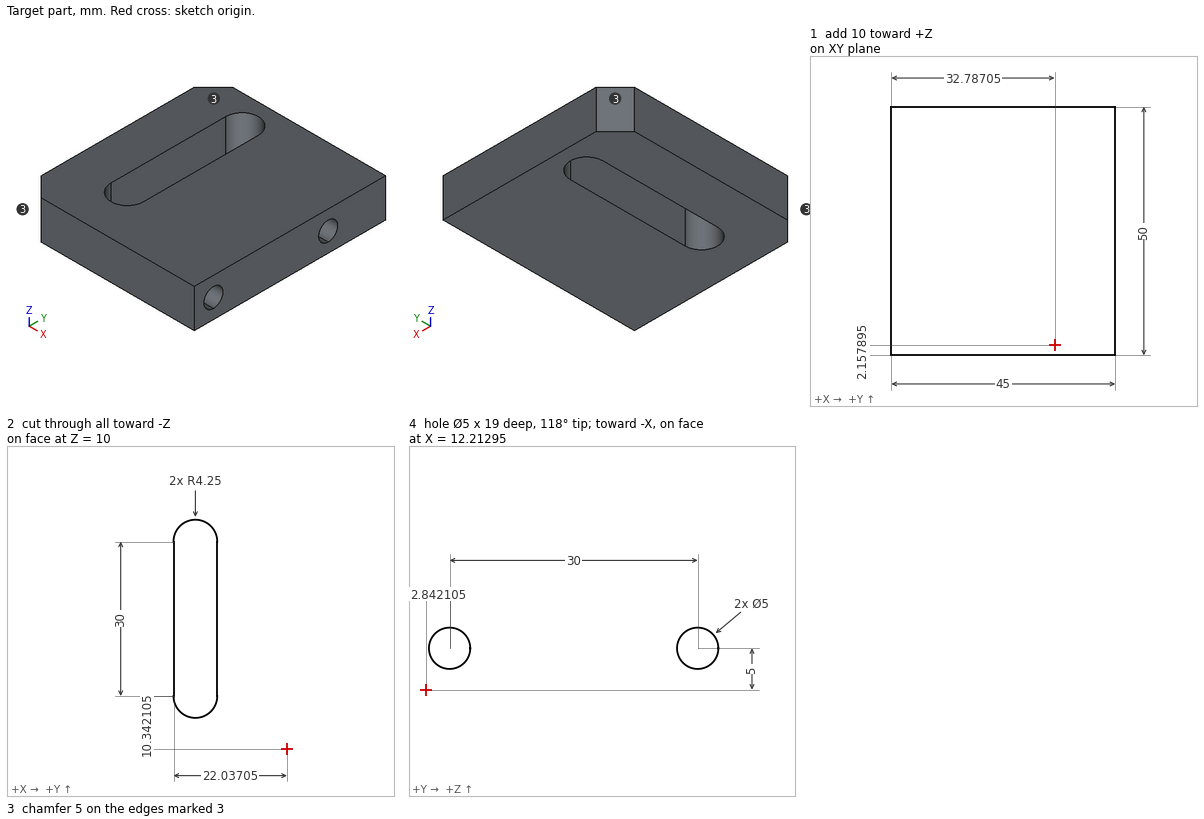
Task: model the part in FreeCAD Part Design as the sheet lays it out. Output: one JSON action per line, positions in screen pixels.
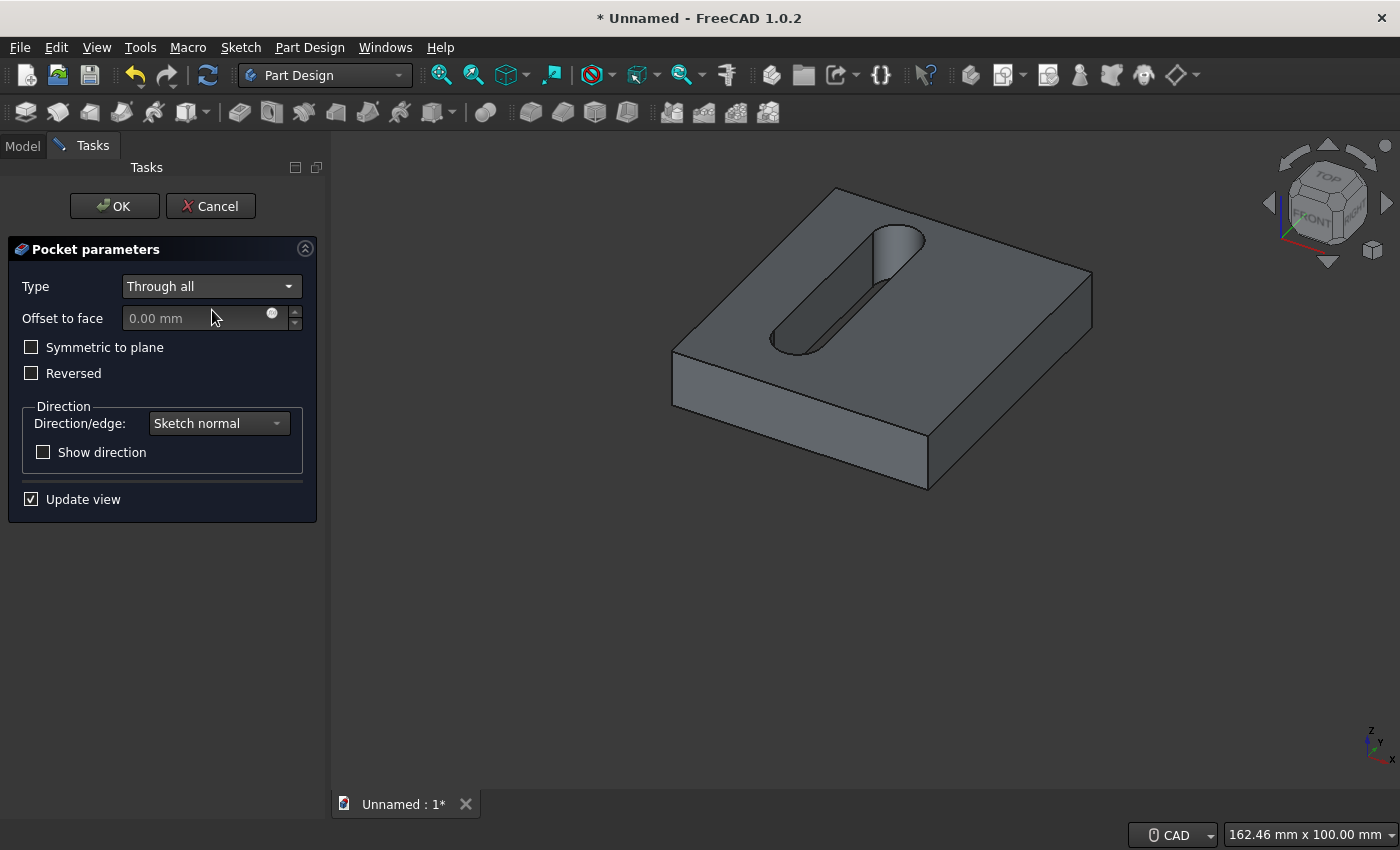
{"action": "left_click", "coordinate": [115, 206]}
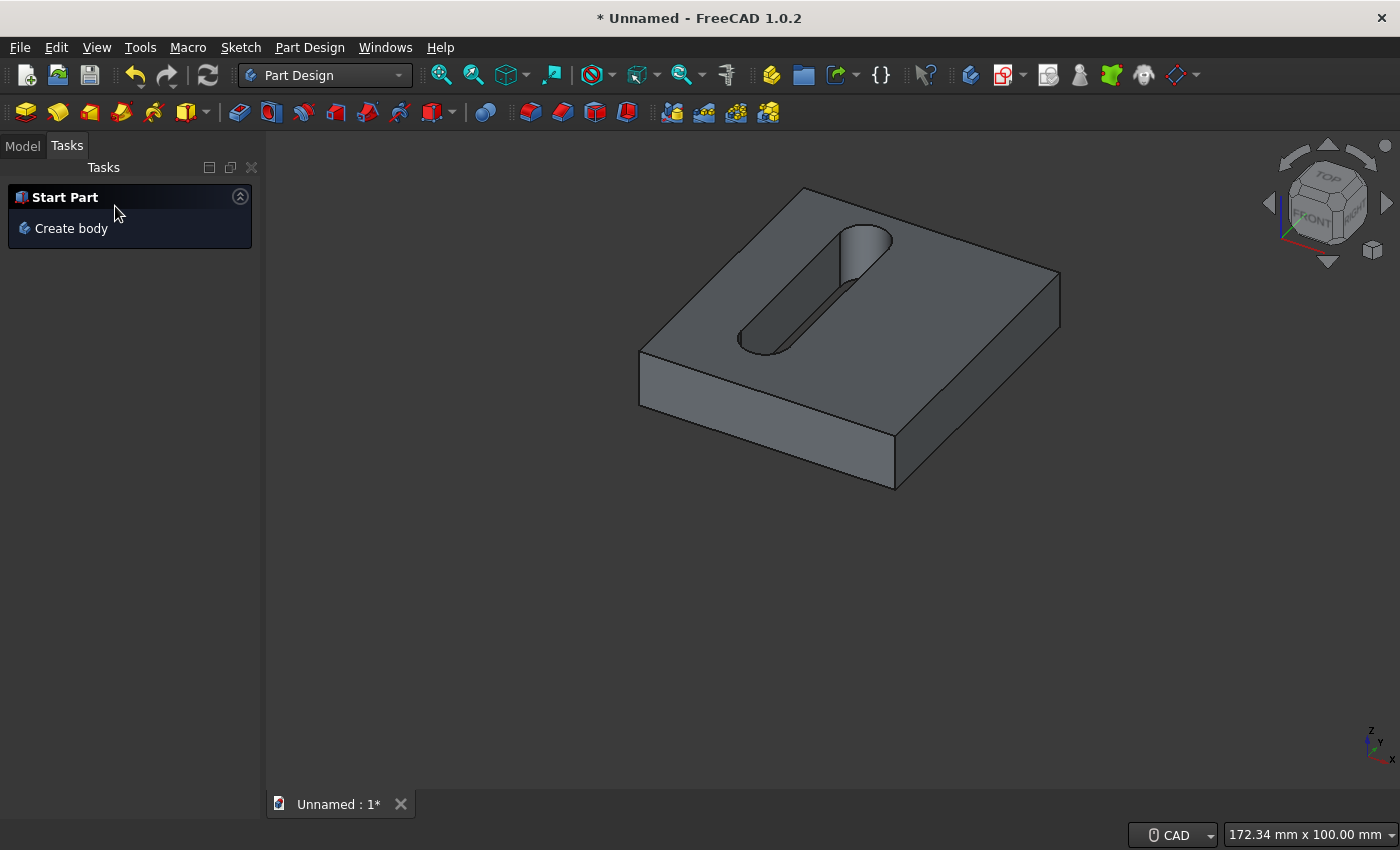
{"action": "key", "text": "0"}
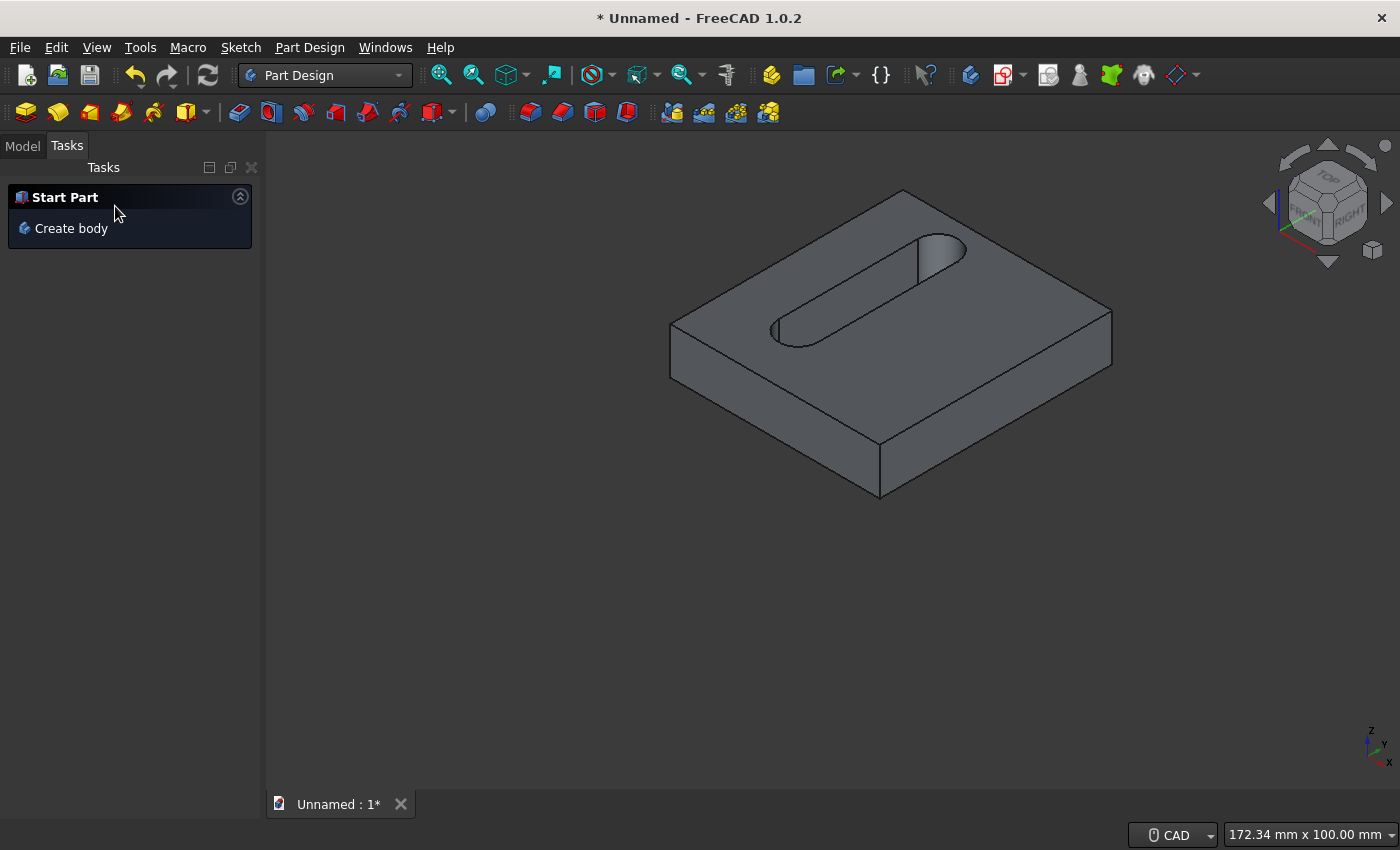
{"action": "key", "text": "2"}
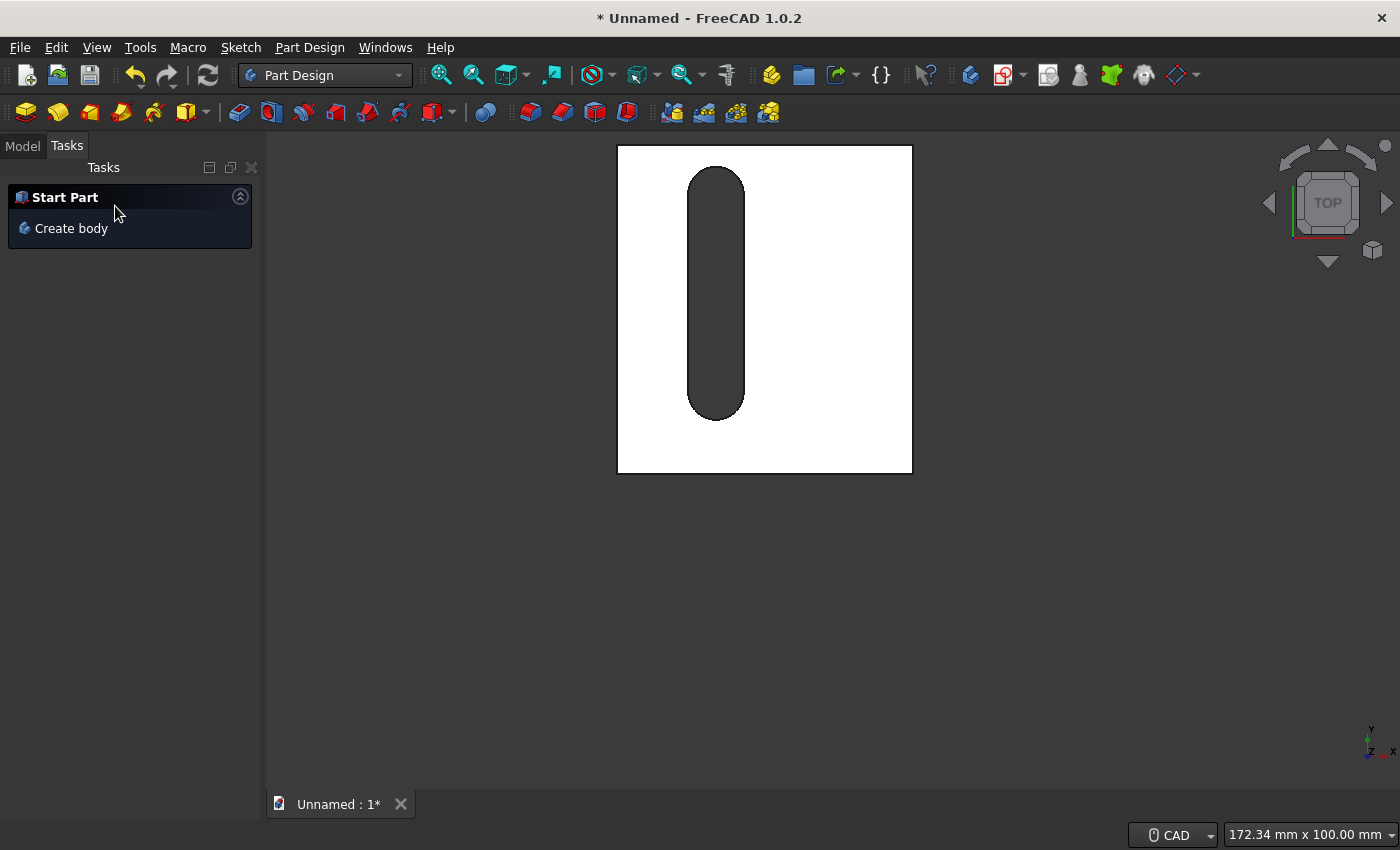
{"action": "key", "text": "1"}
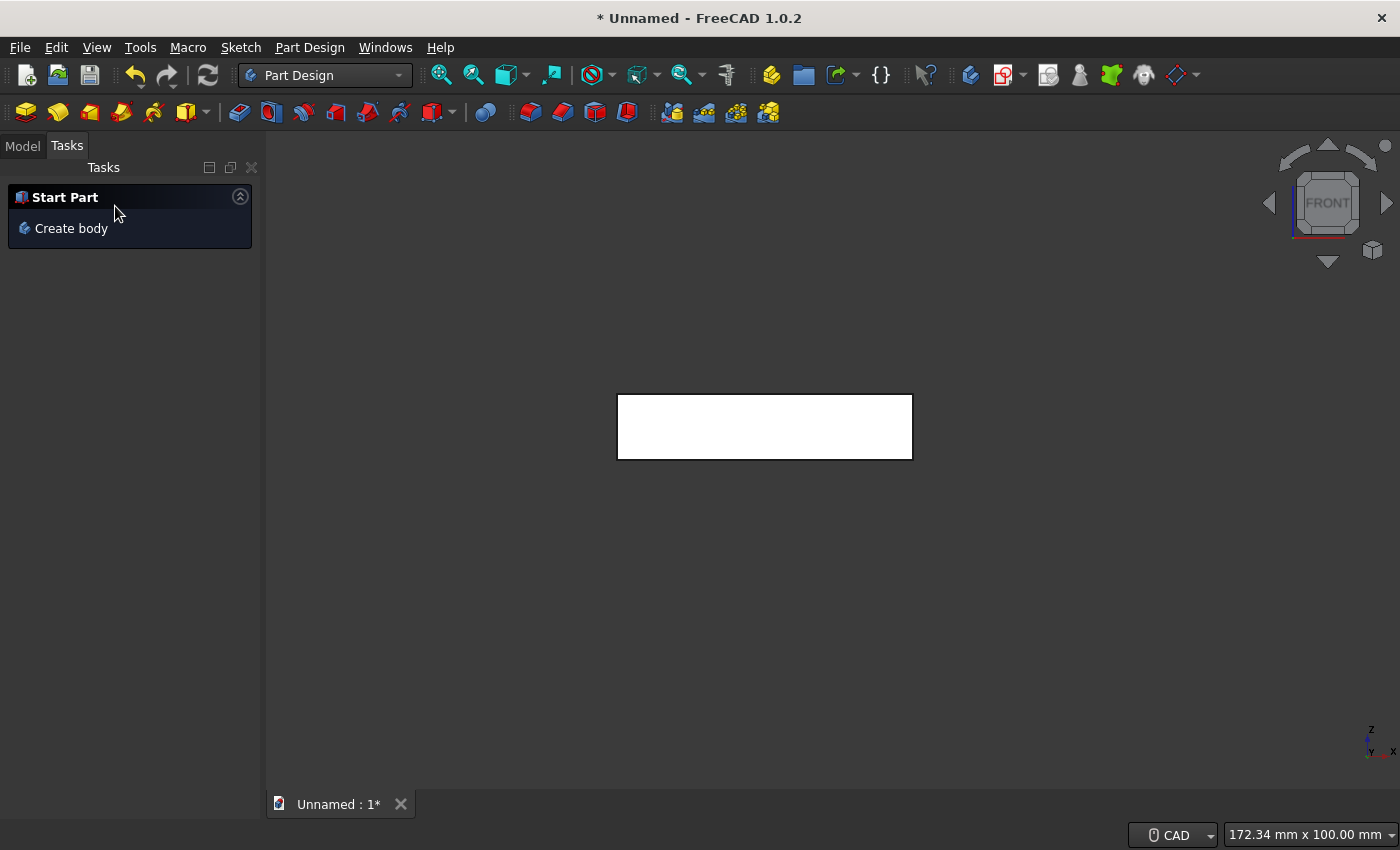
{"action": "left_click", "coordinate": [442, 76]}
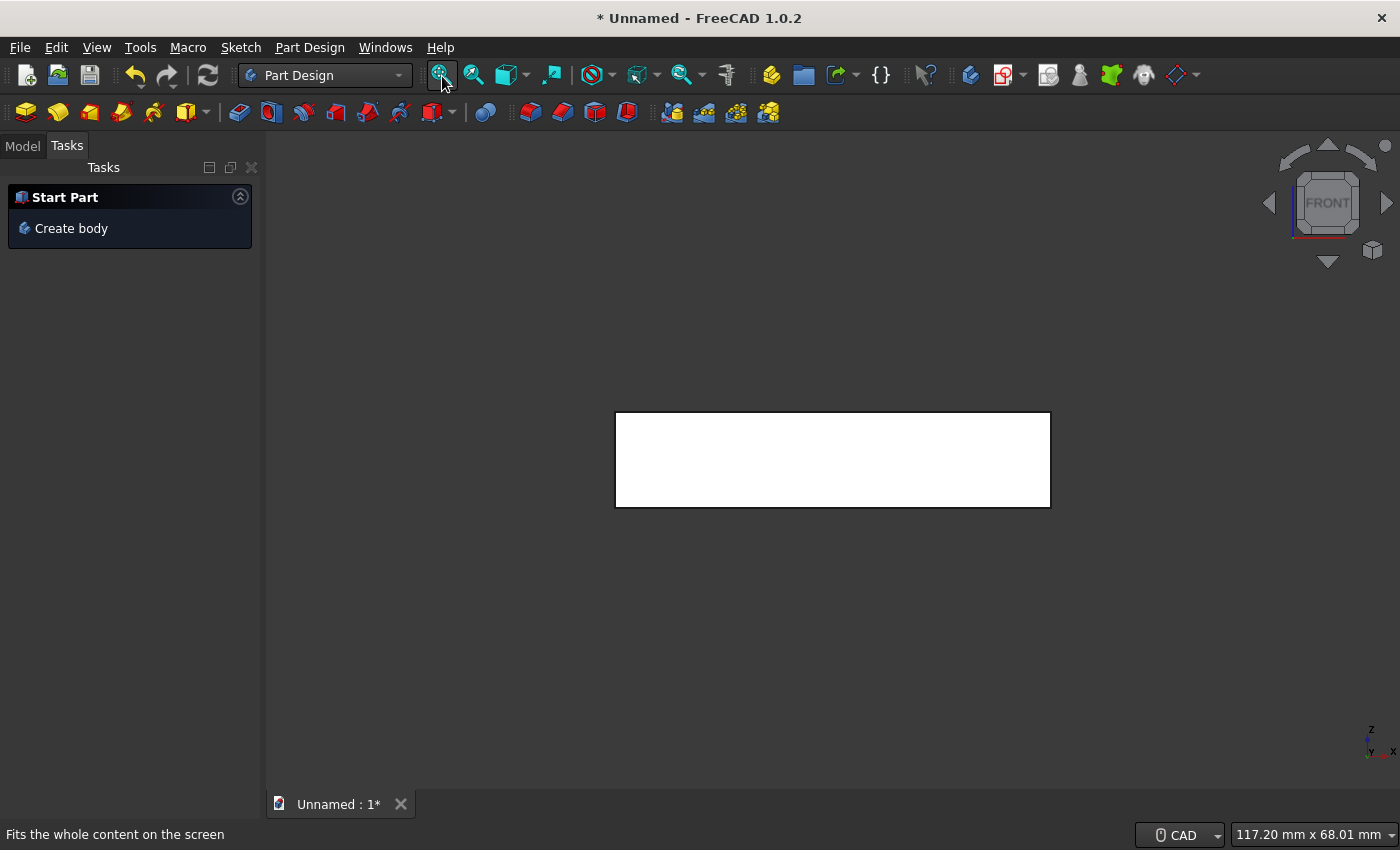
{"action": "left_click", "coordinate": [615, 459]}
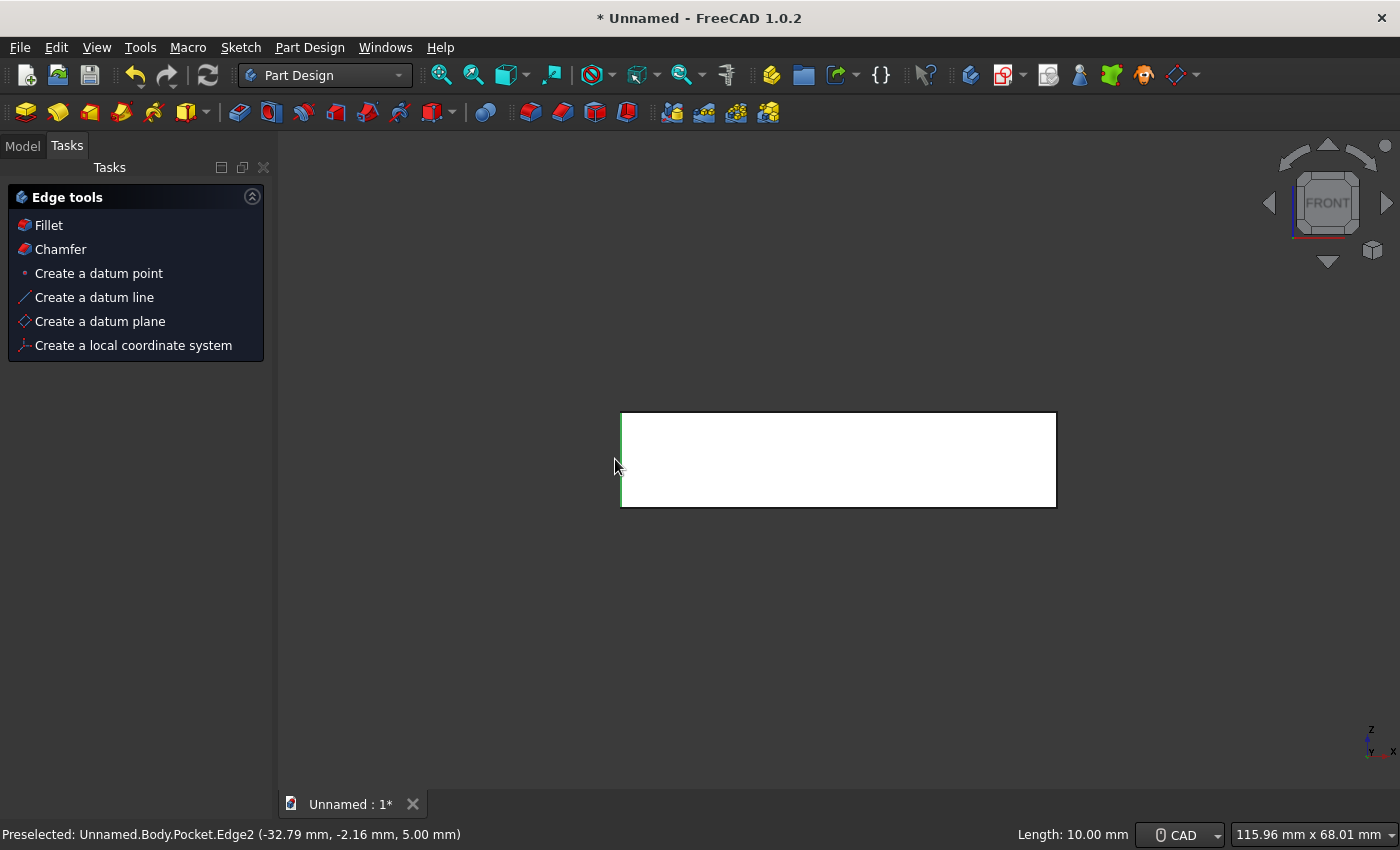
{"action": "key", "text": "3"}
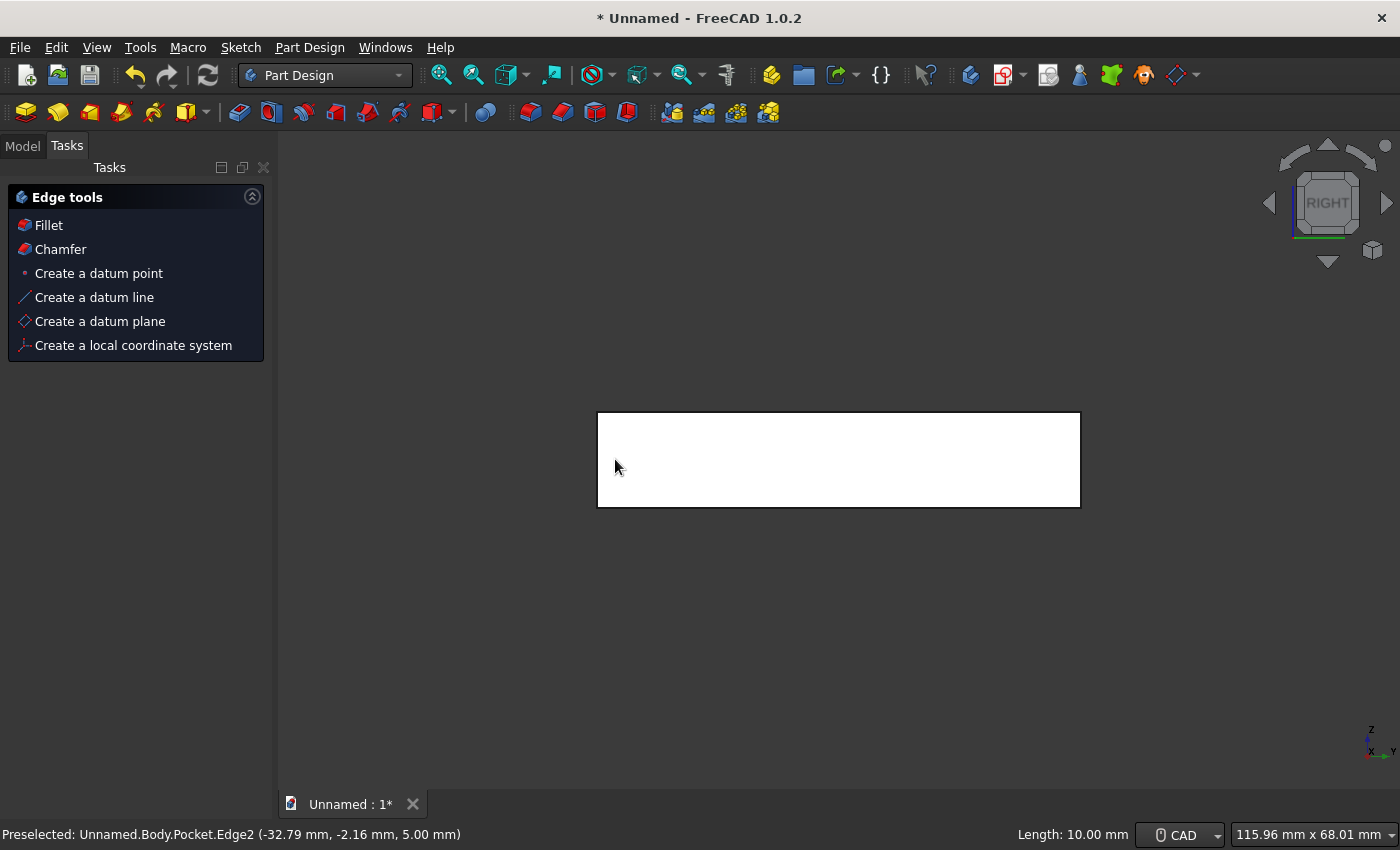
{"action": "left_click", "coordinate": [442, 76]}